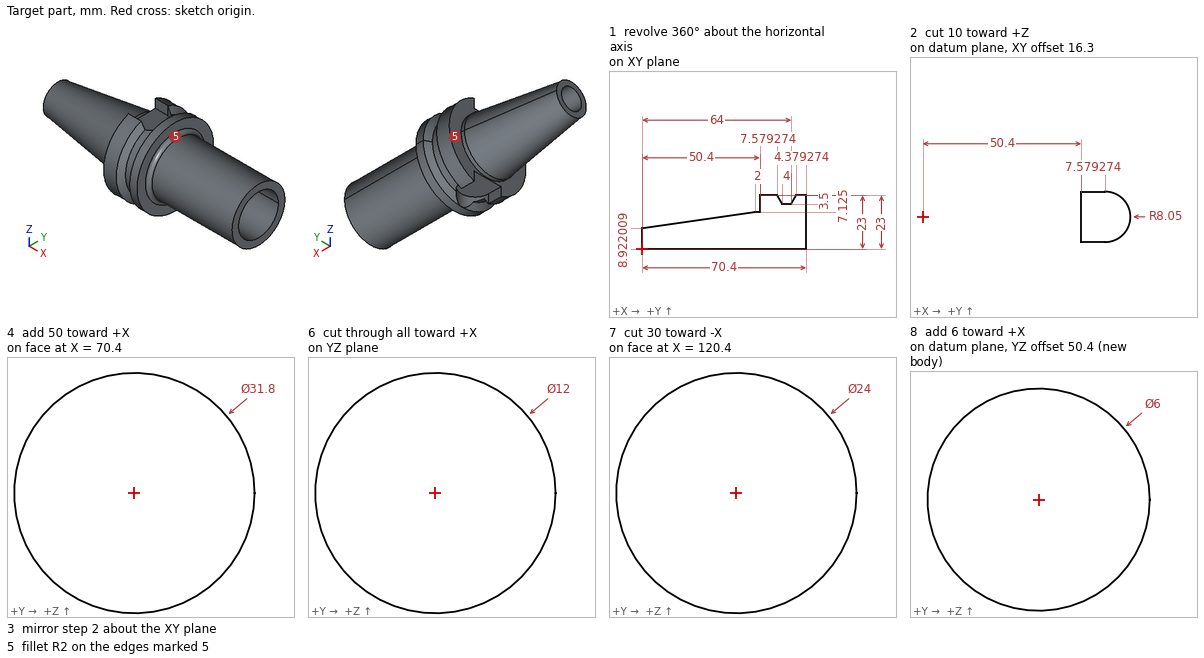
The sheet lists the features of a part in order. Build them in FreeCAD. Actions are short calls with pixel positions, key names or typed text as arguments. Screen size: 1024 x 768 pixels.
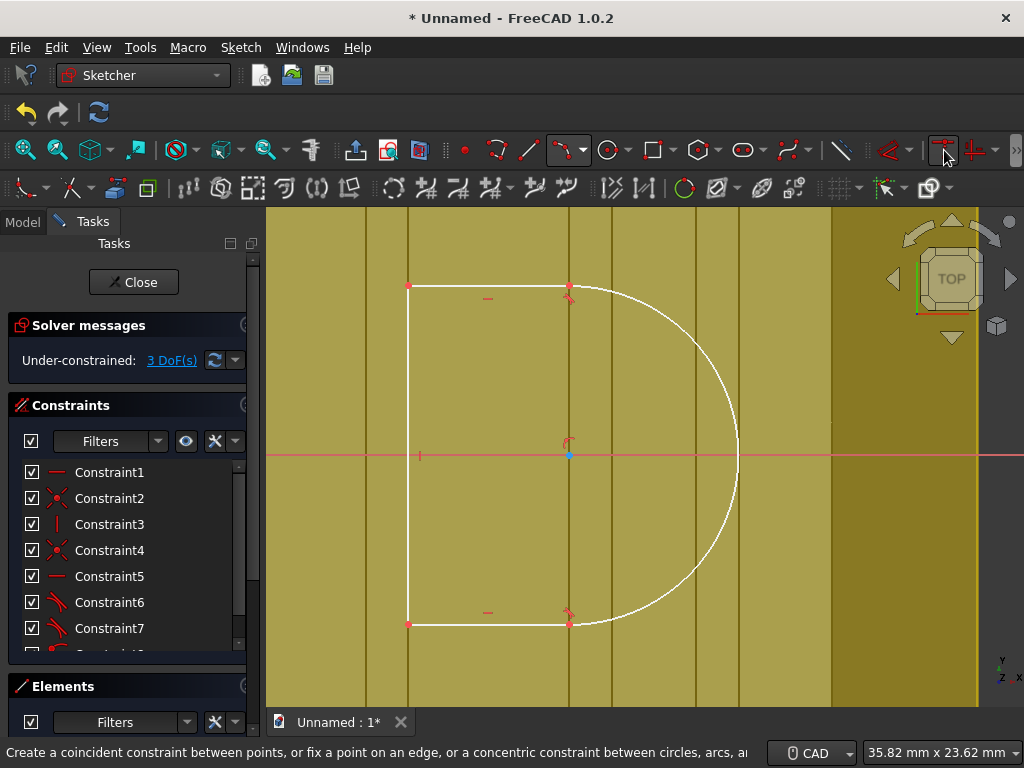
click(706, 555)
click(732, 574)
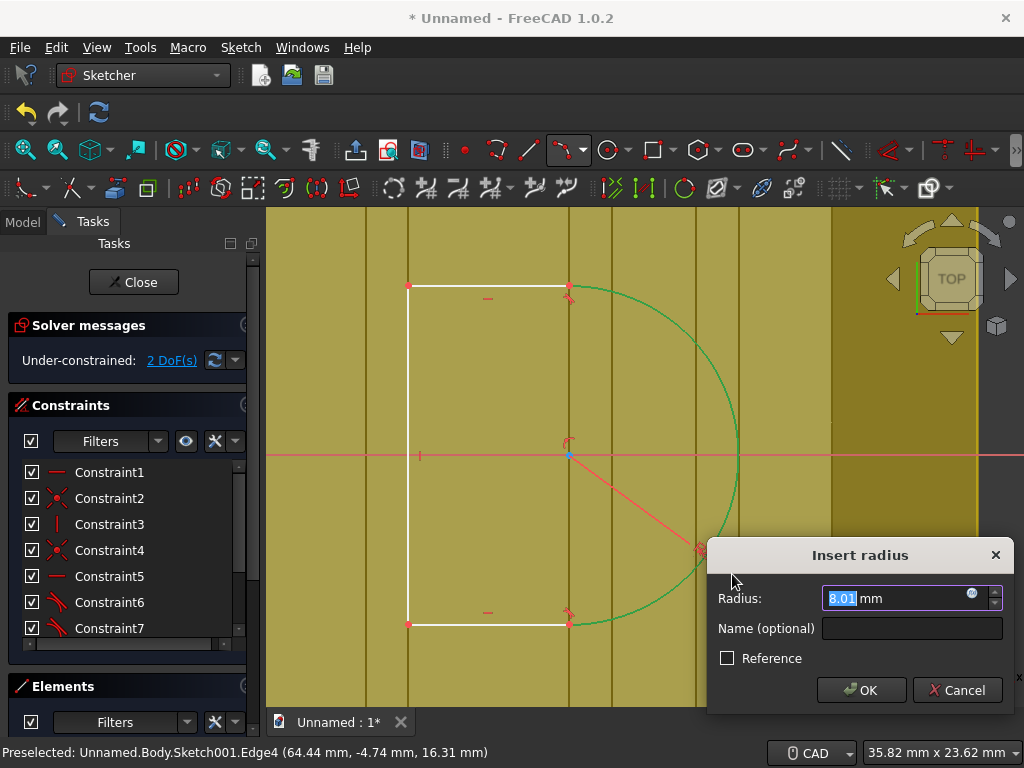
text(8.05)
key(Return)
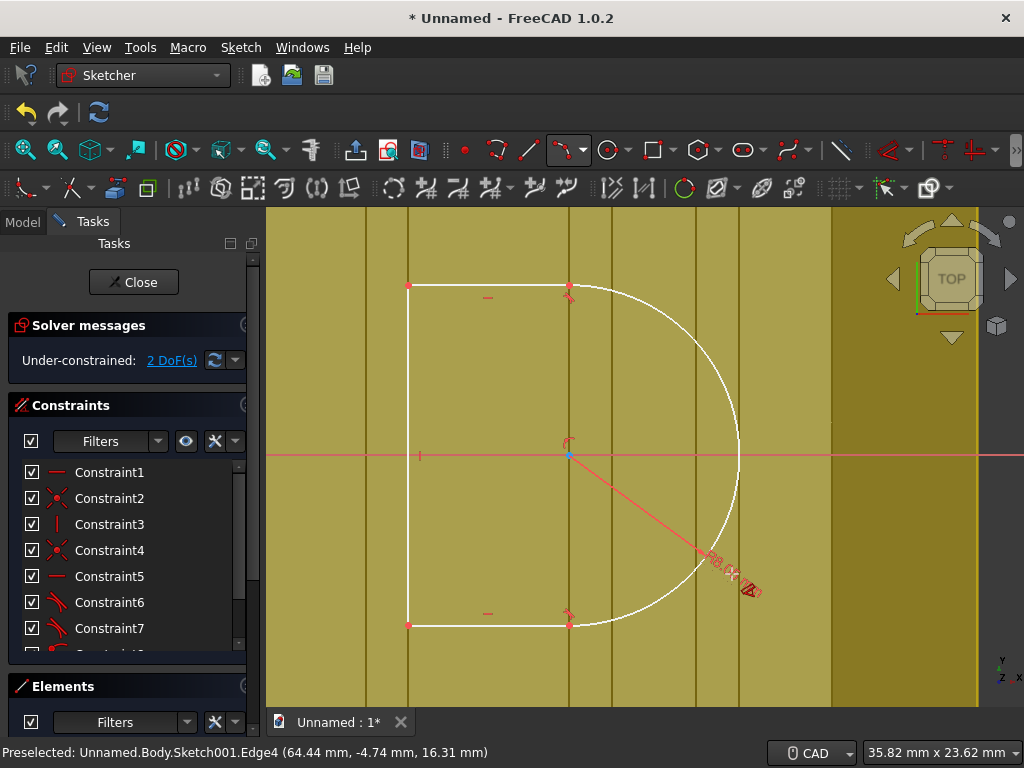
click(408, 285)
click(351, 251)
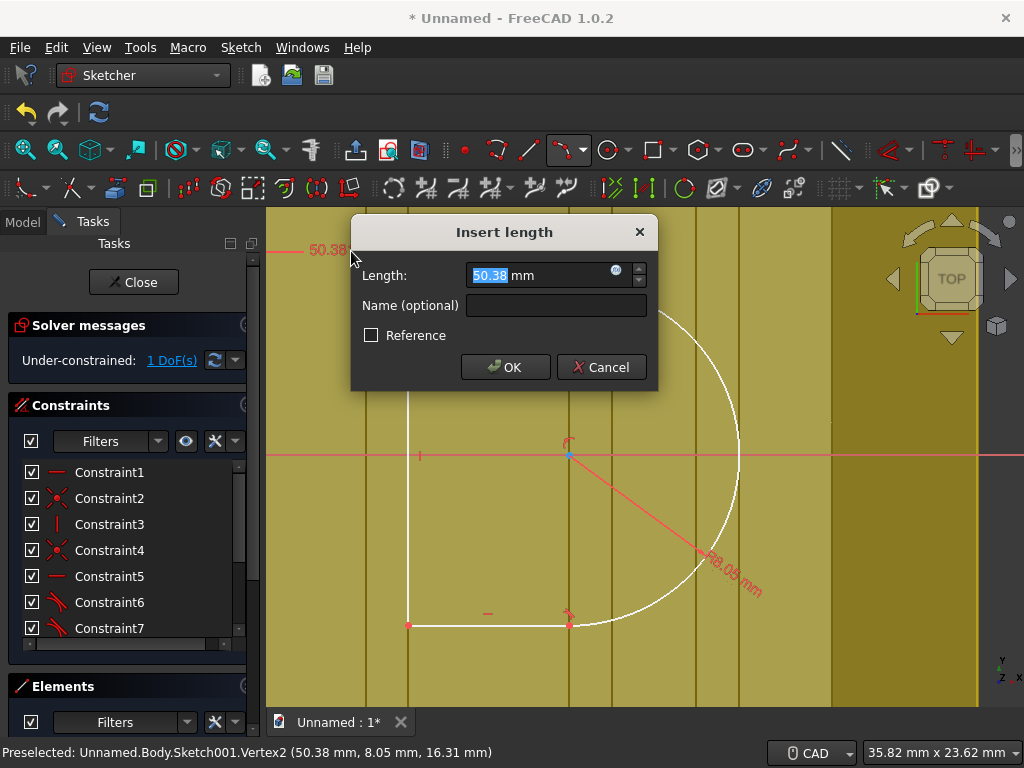
text(50.4)
key(Return)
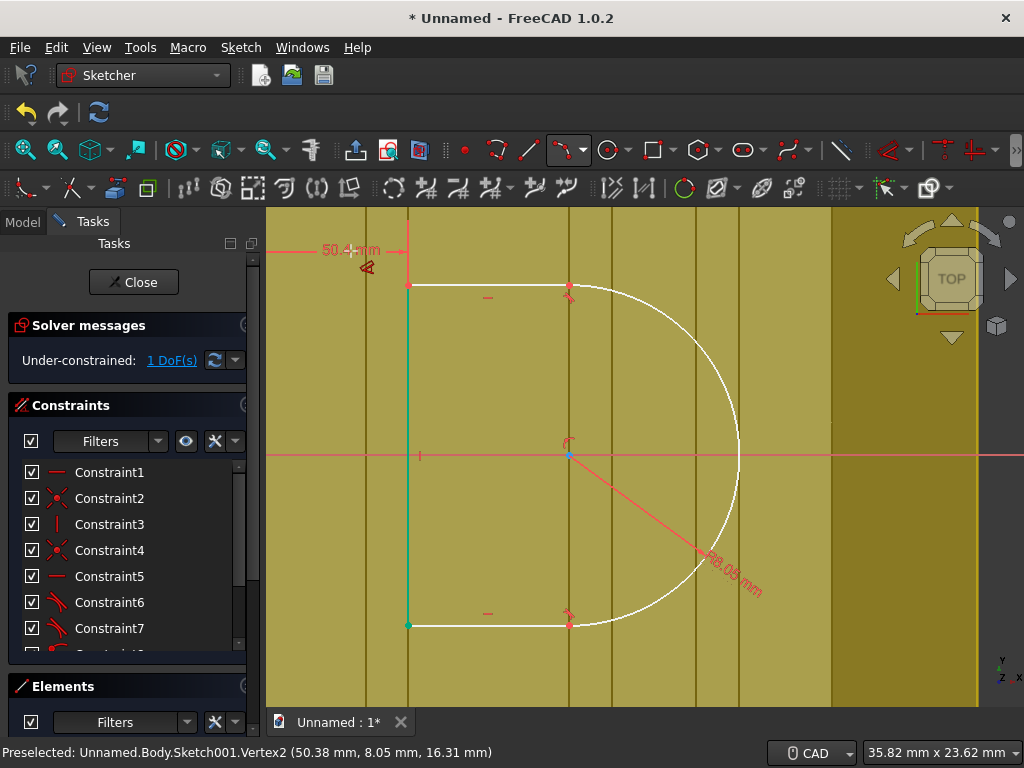
click(521, 285)
click(489, 251)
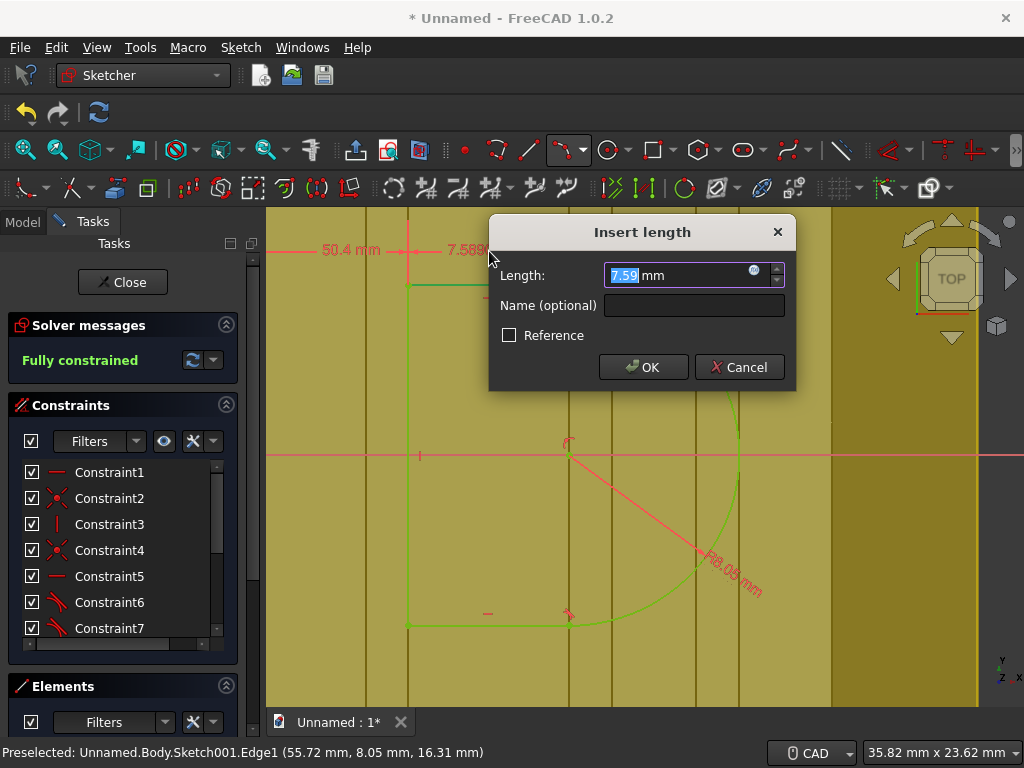
text(7.579274)
key(Return)
key(Escape)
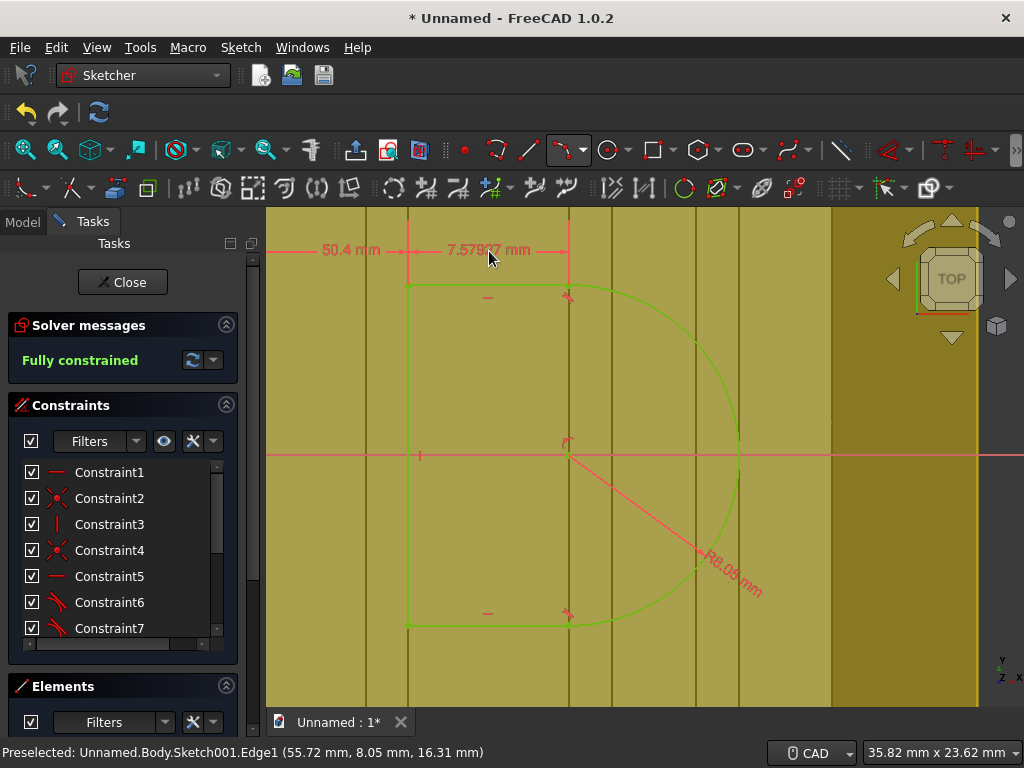
click(123, 282)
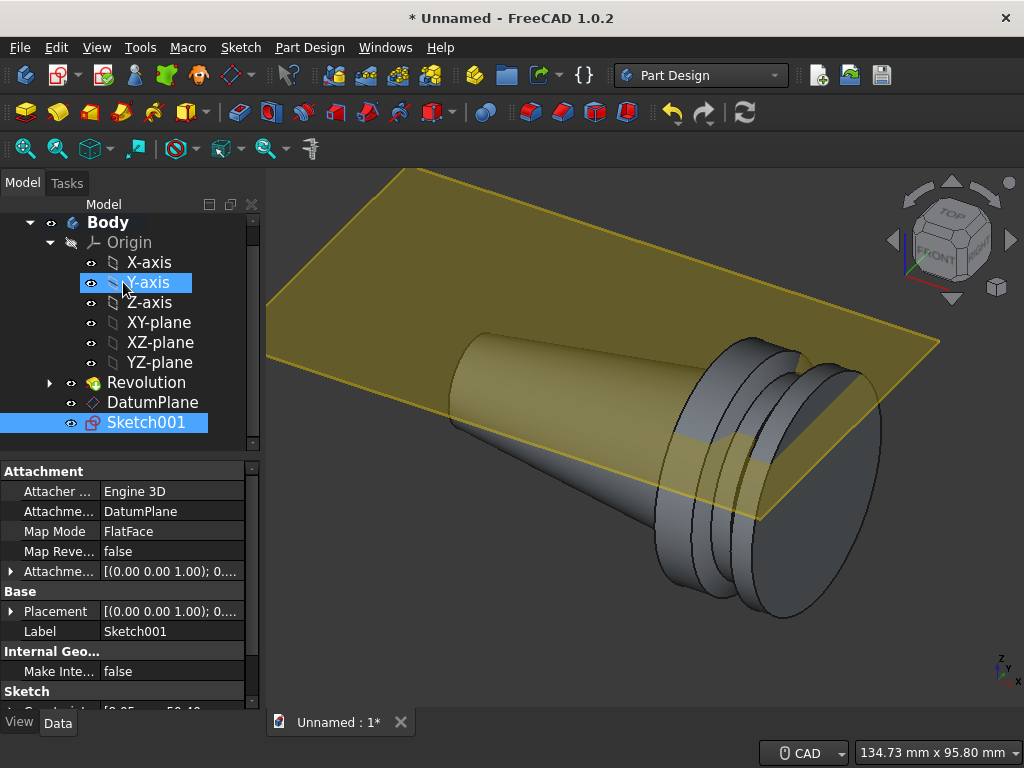
click(240, 112)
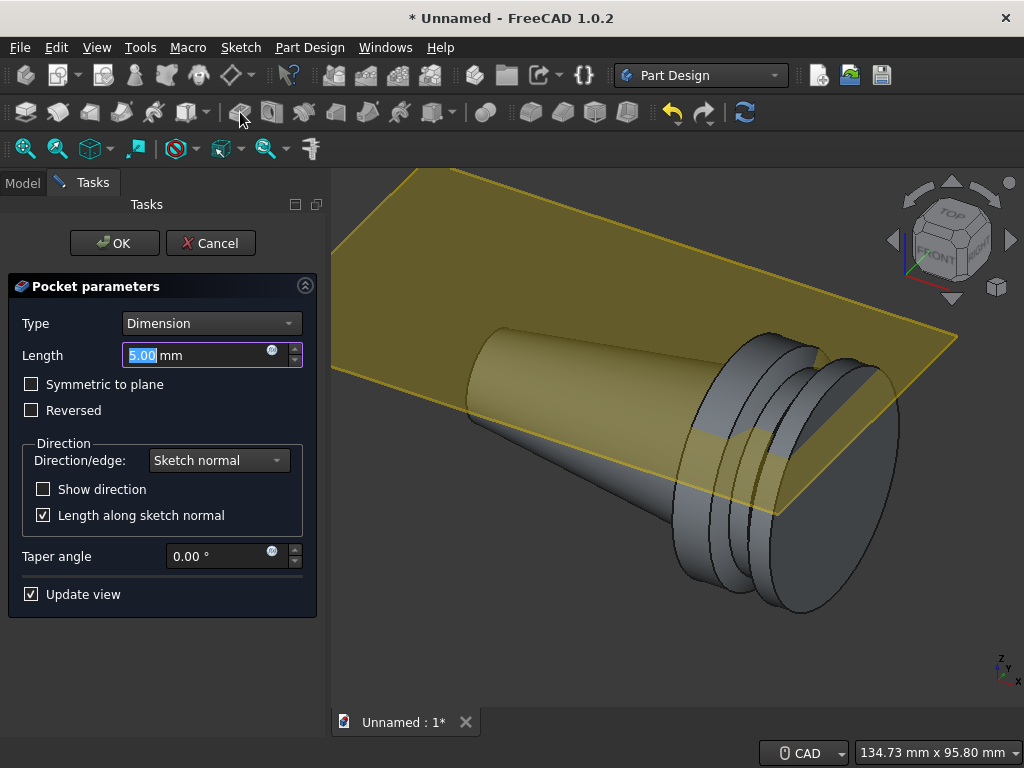
text(10)
key(Tab)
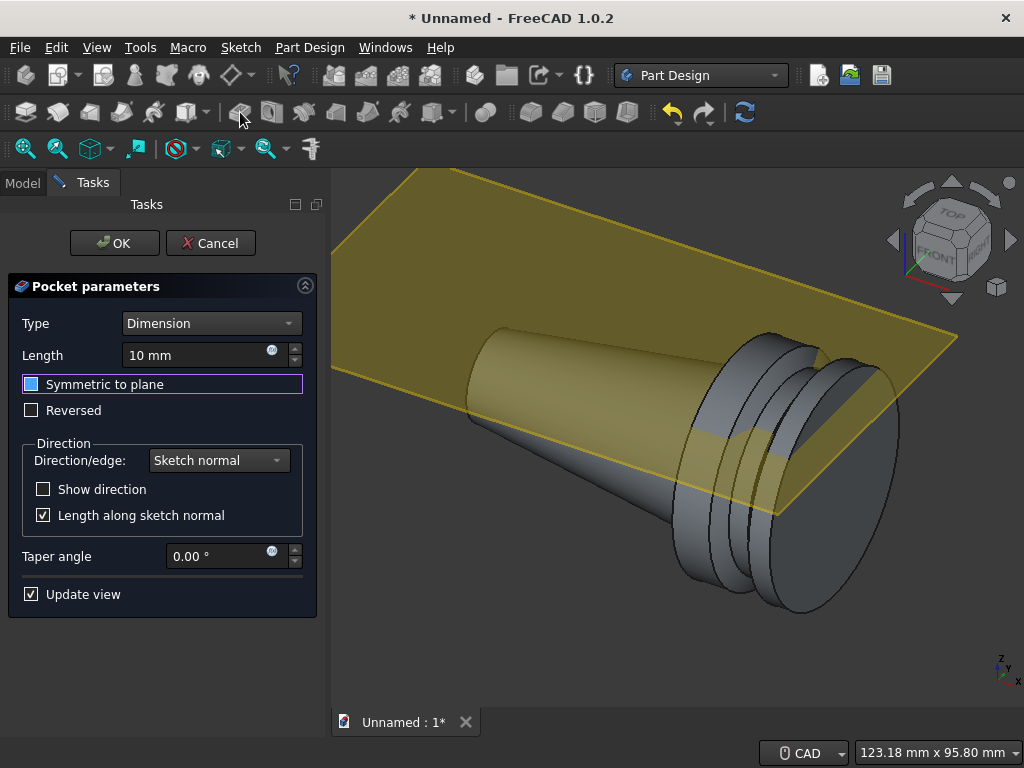
click(30, 410)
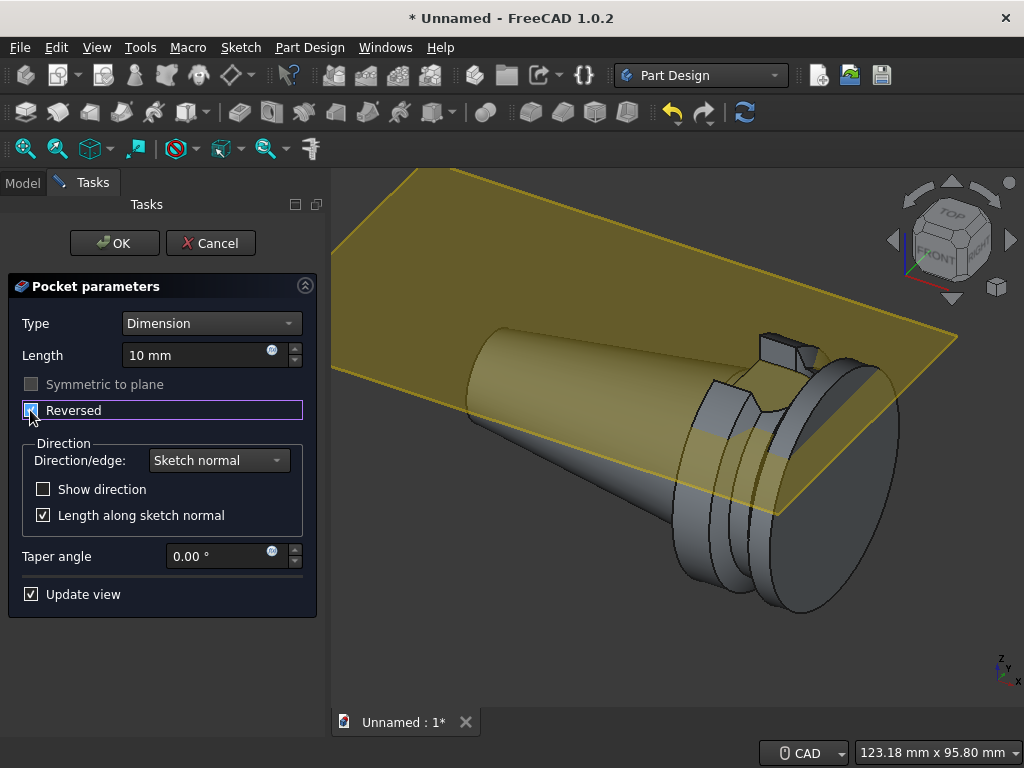
click(115, 243)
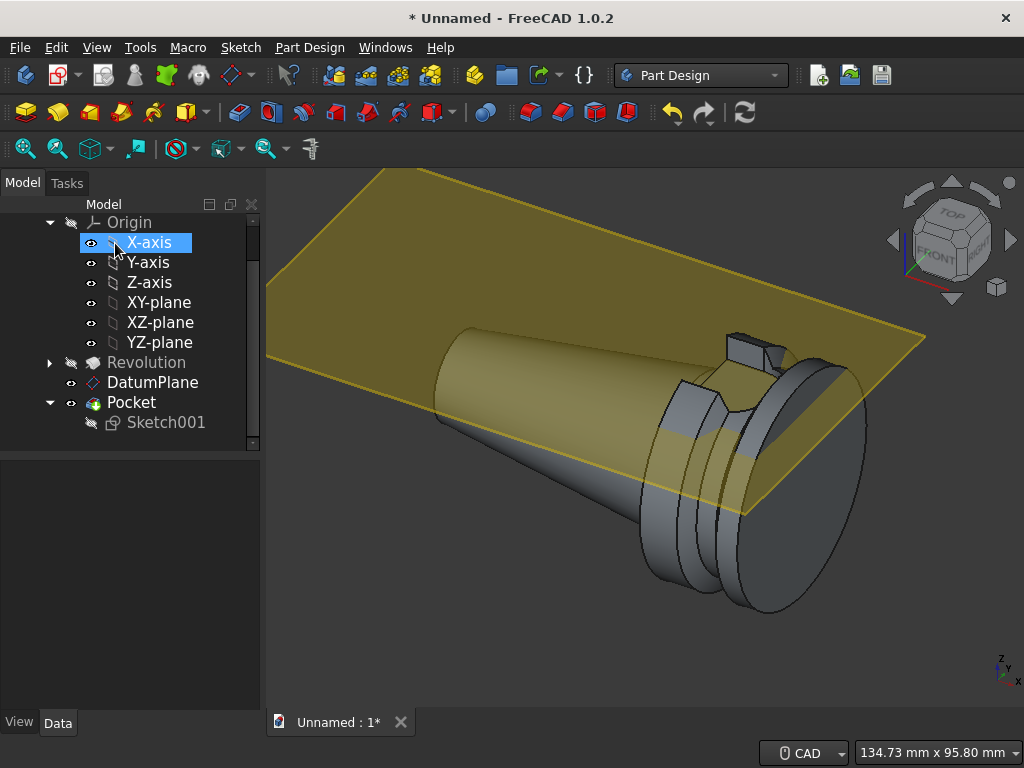
click(116, 383)
key(space)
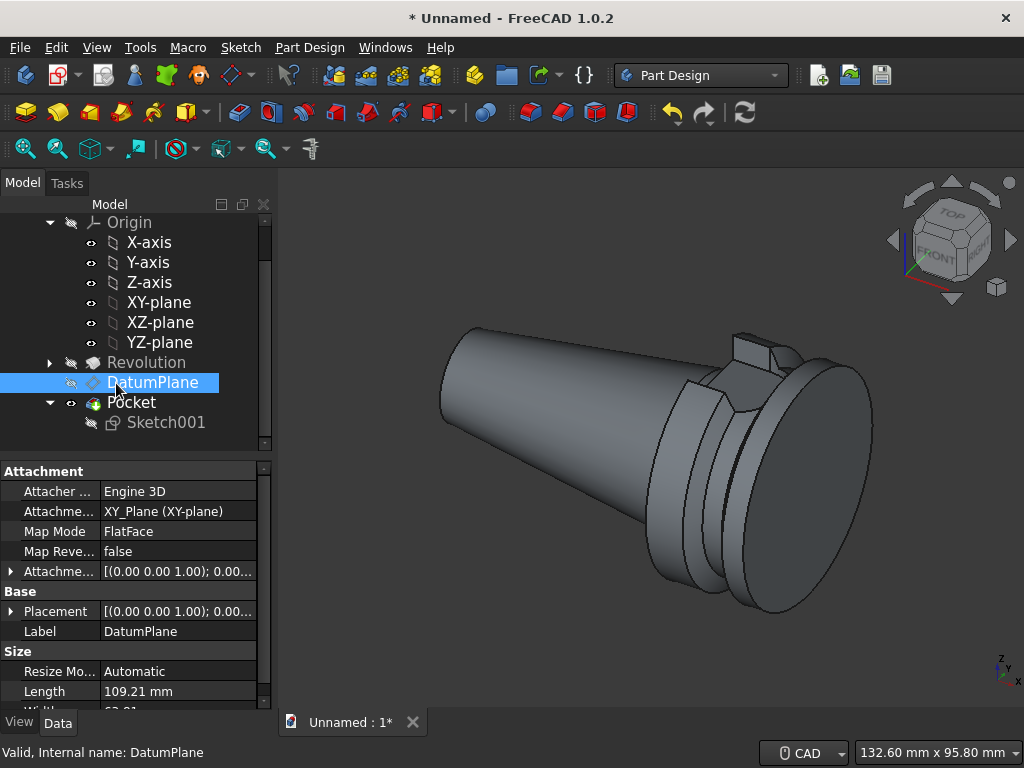
click(116, 403)